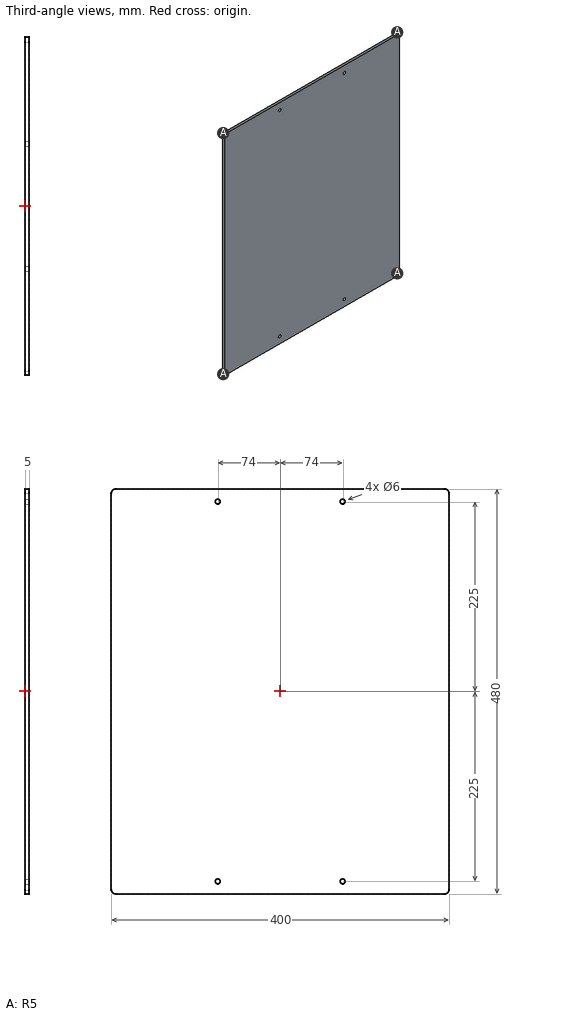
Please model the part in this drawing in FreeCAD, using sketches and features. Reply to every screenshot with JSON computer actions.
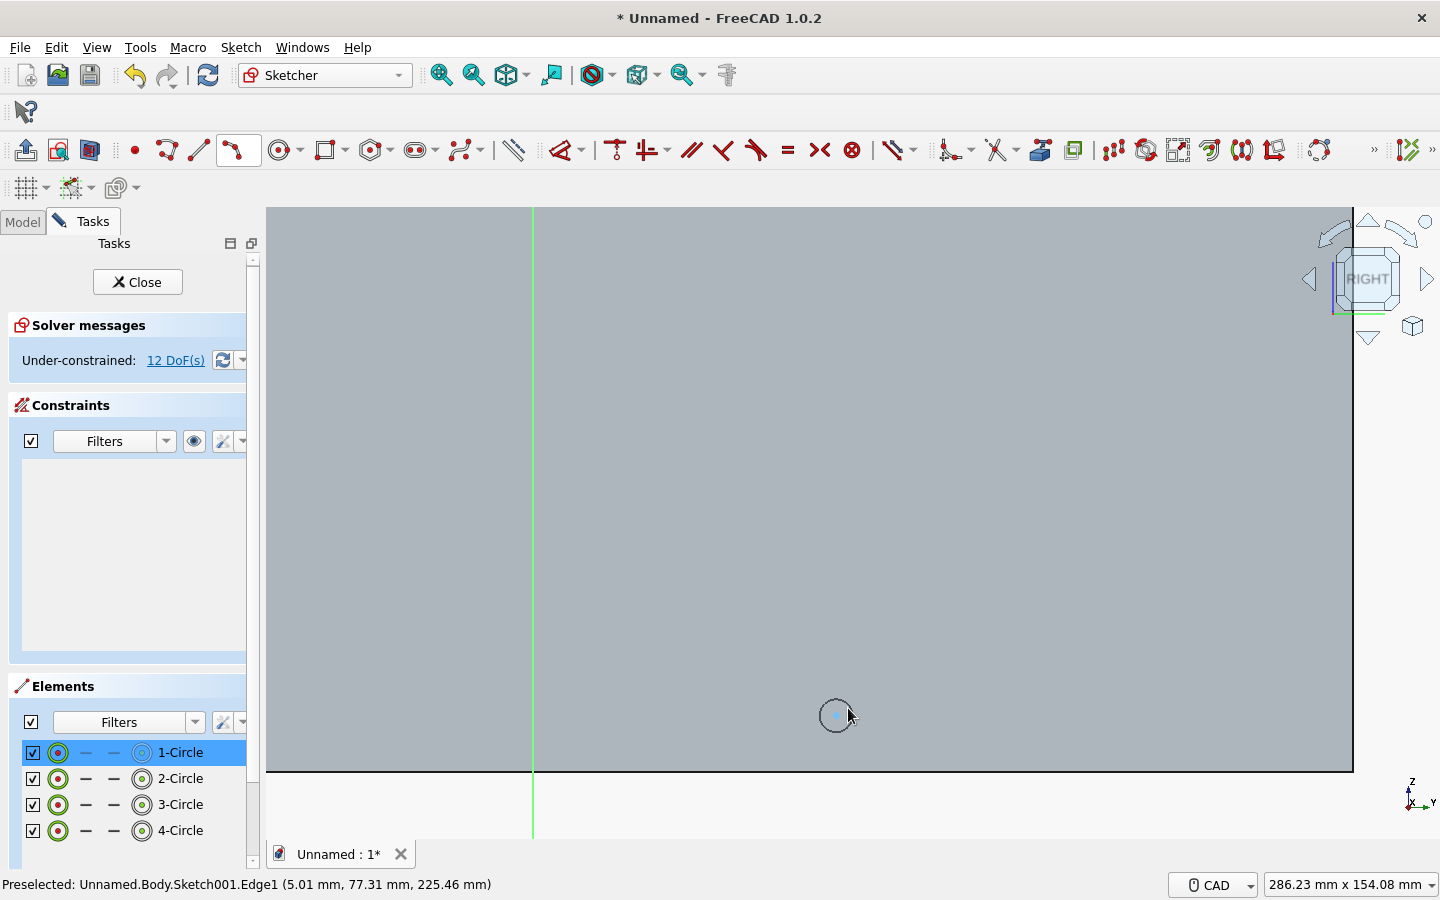
{"action": "left_click", "coordinate": [848, 704]}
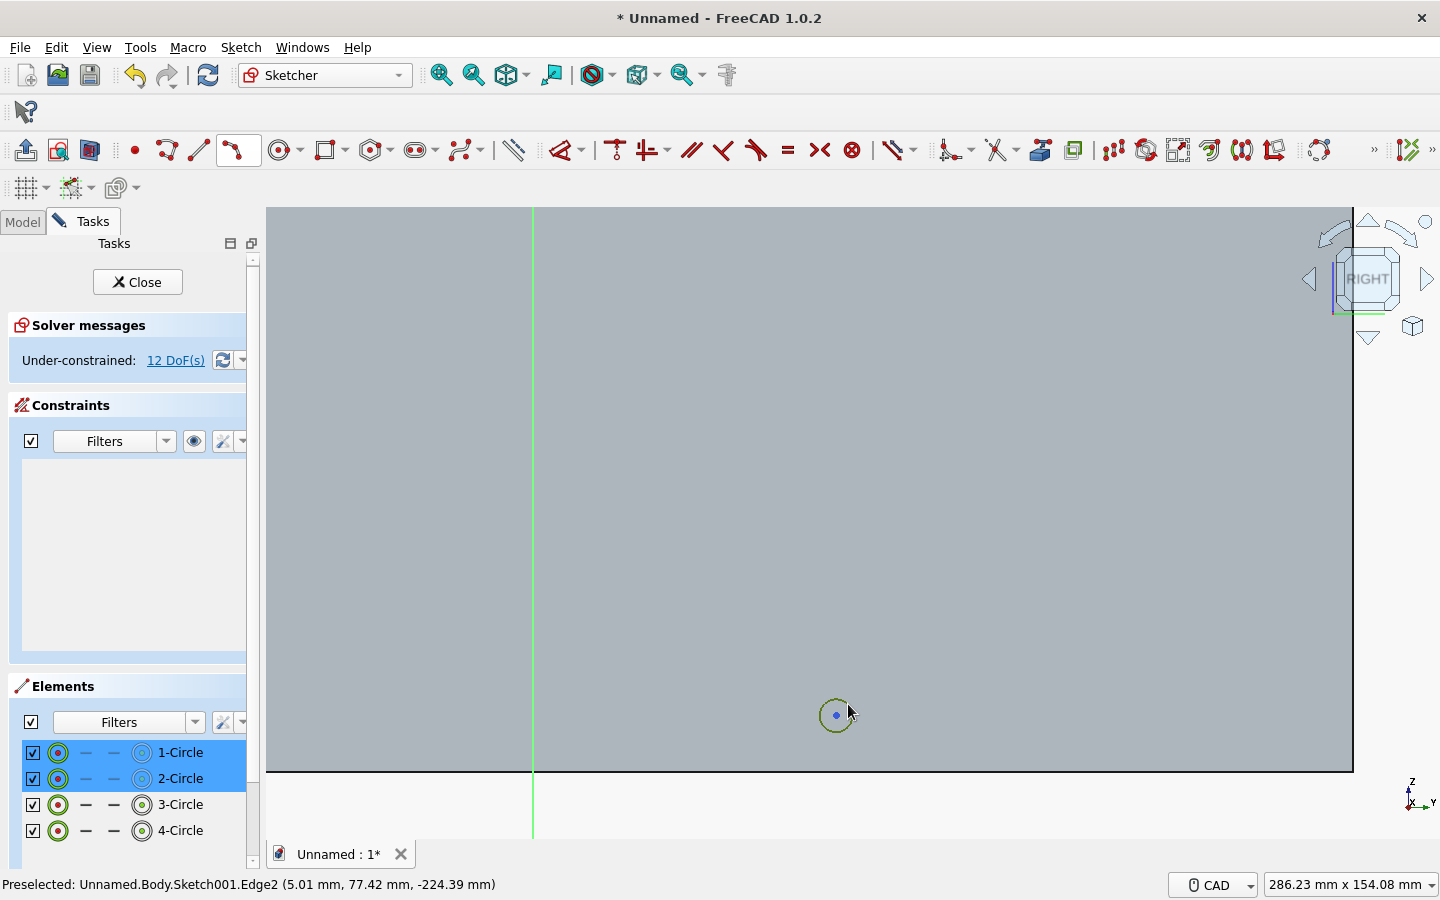
{"action": "scroll", "coordinate": [848, 709], "scroll_direction": "down", "scroll_amount": 8}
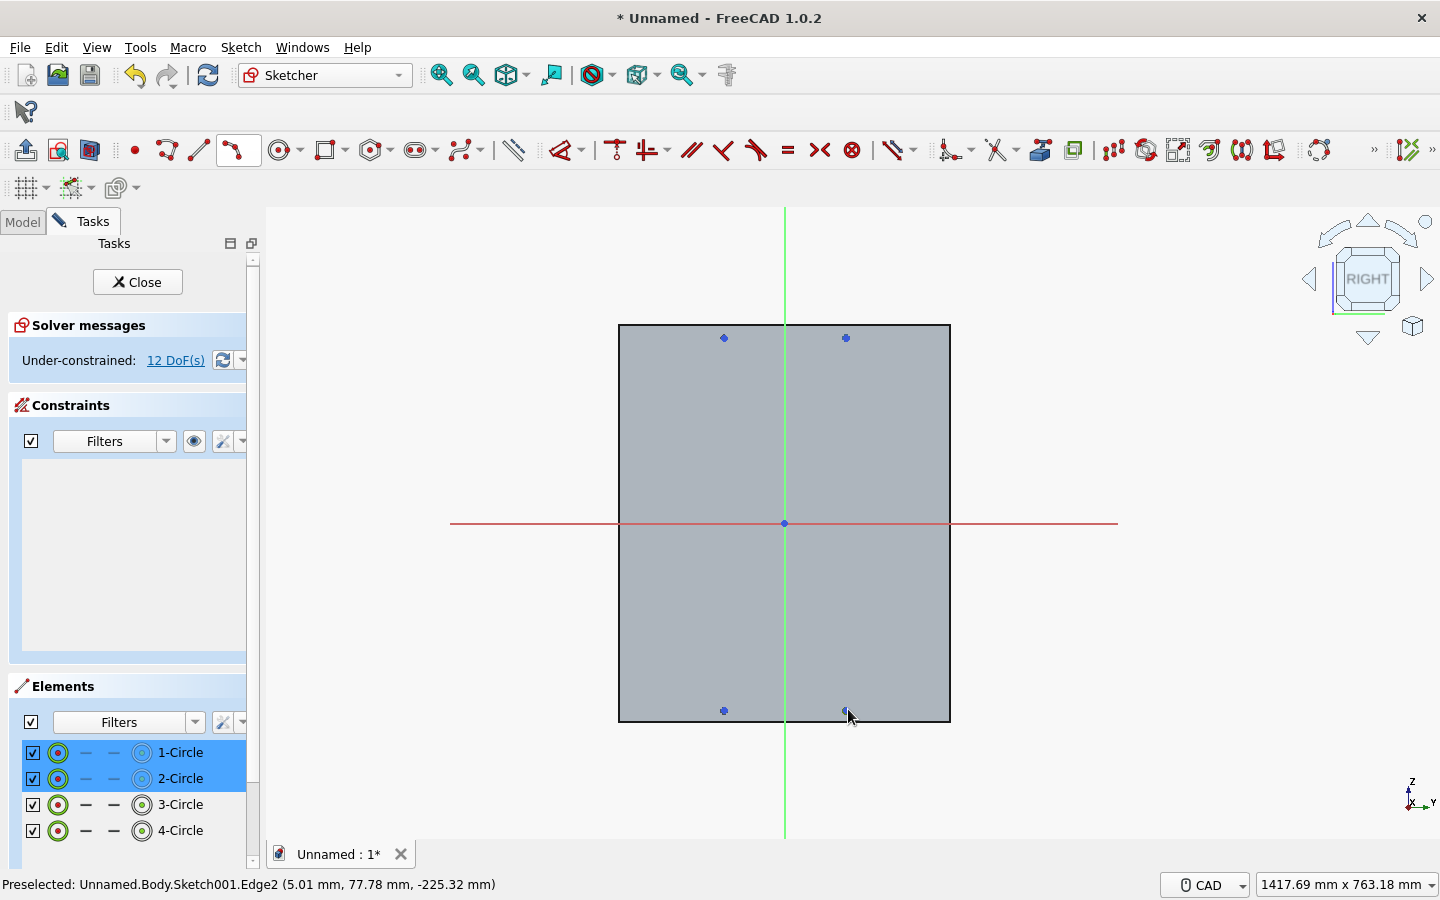
{"action": "scroll", "coordinate": [726, 336], "scroll_direction": "up", "scroll_amount": 9}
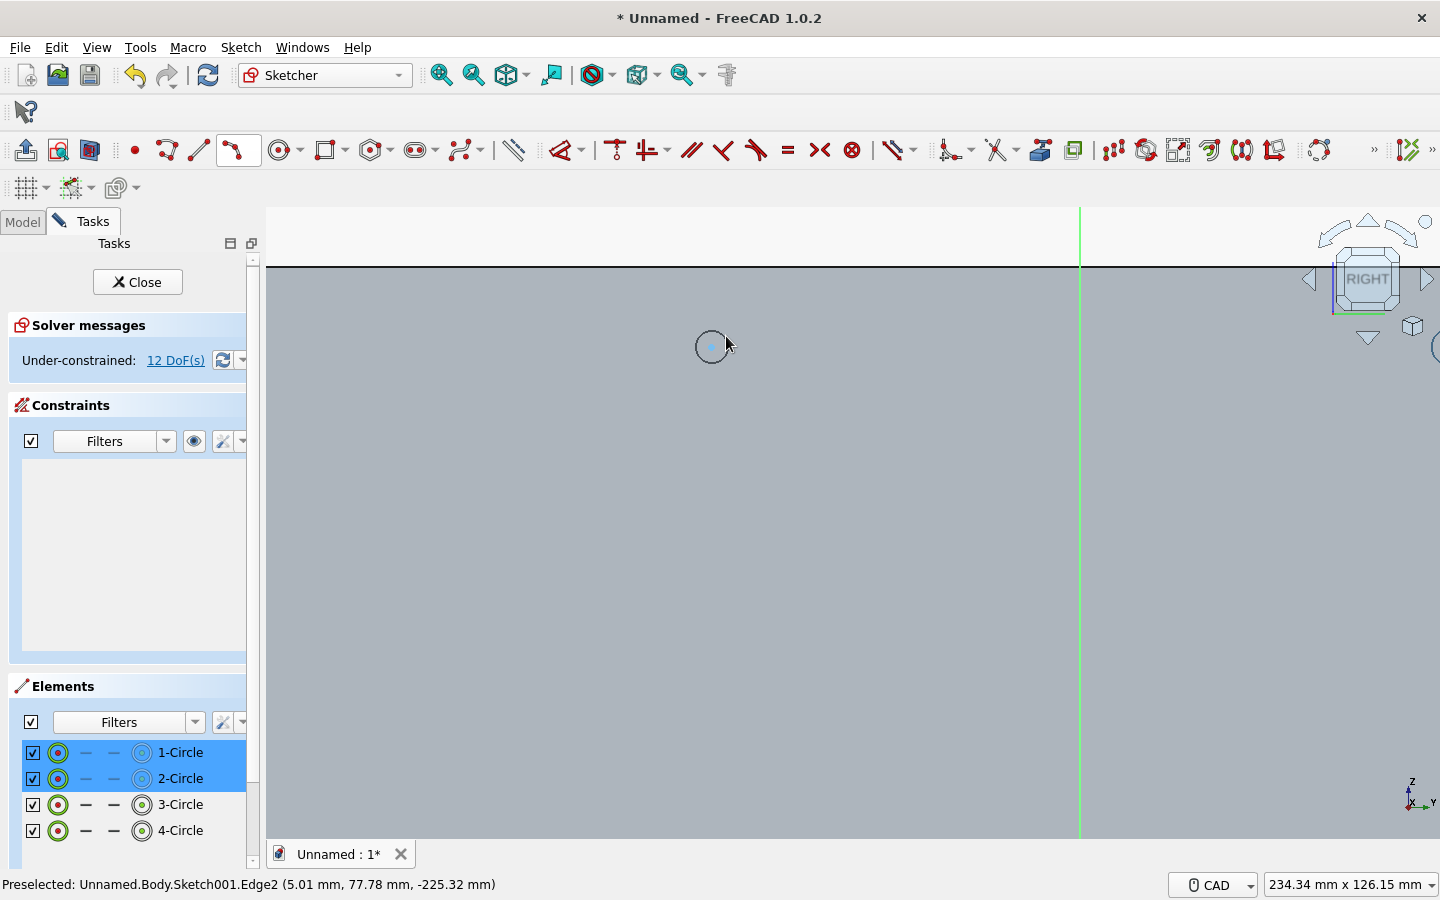
{"action": "left_click", "coordinate": [723, 336]}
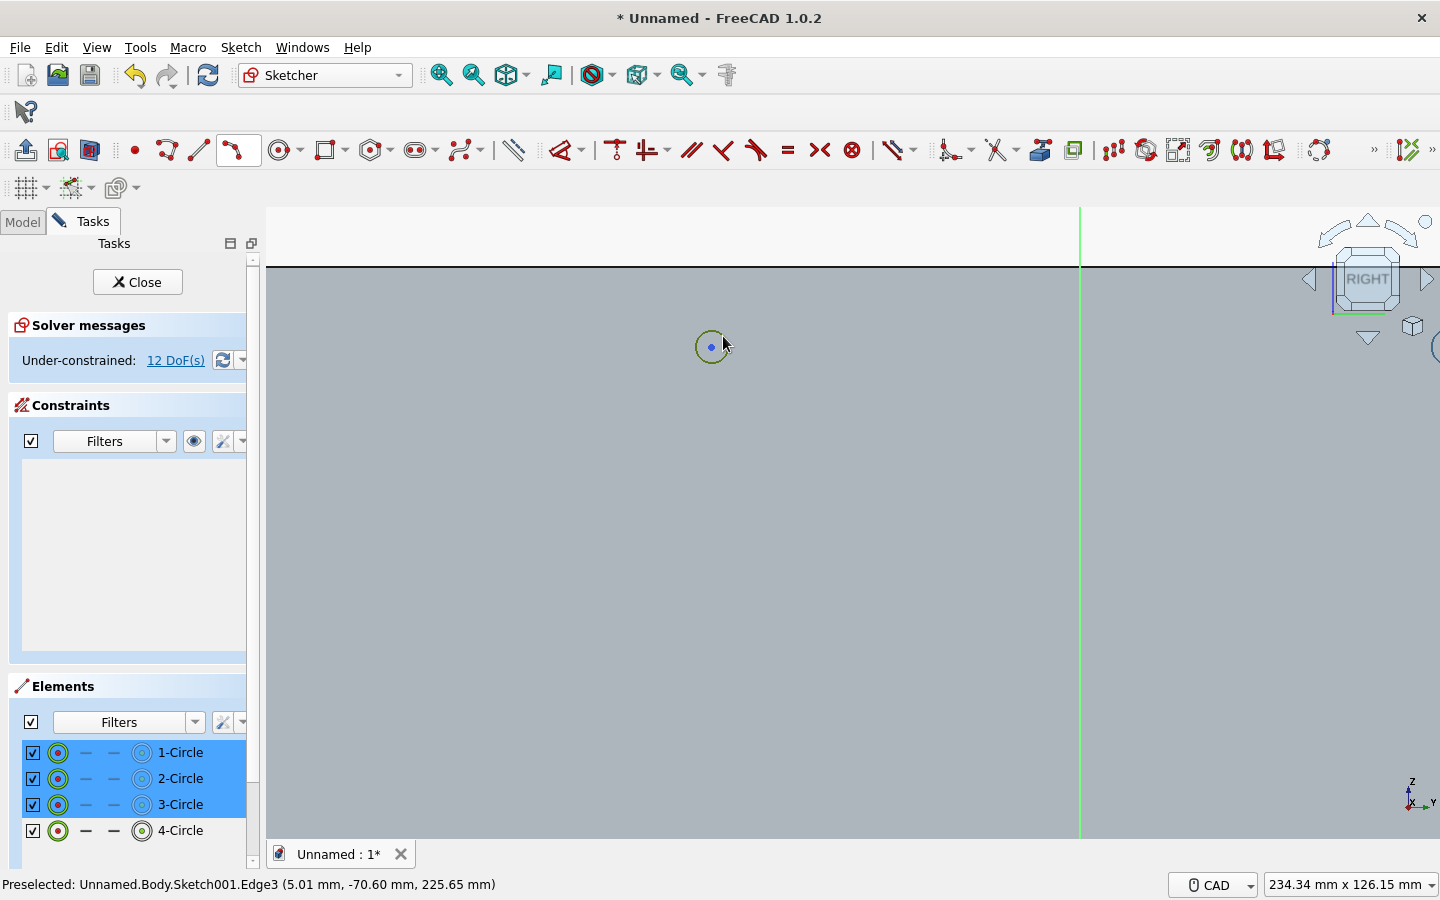
{"action": "scroll", "coordinate": [726, 335], "scroll_direction": "down", "scroll_amount": 9}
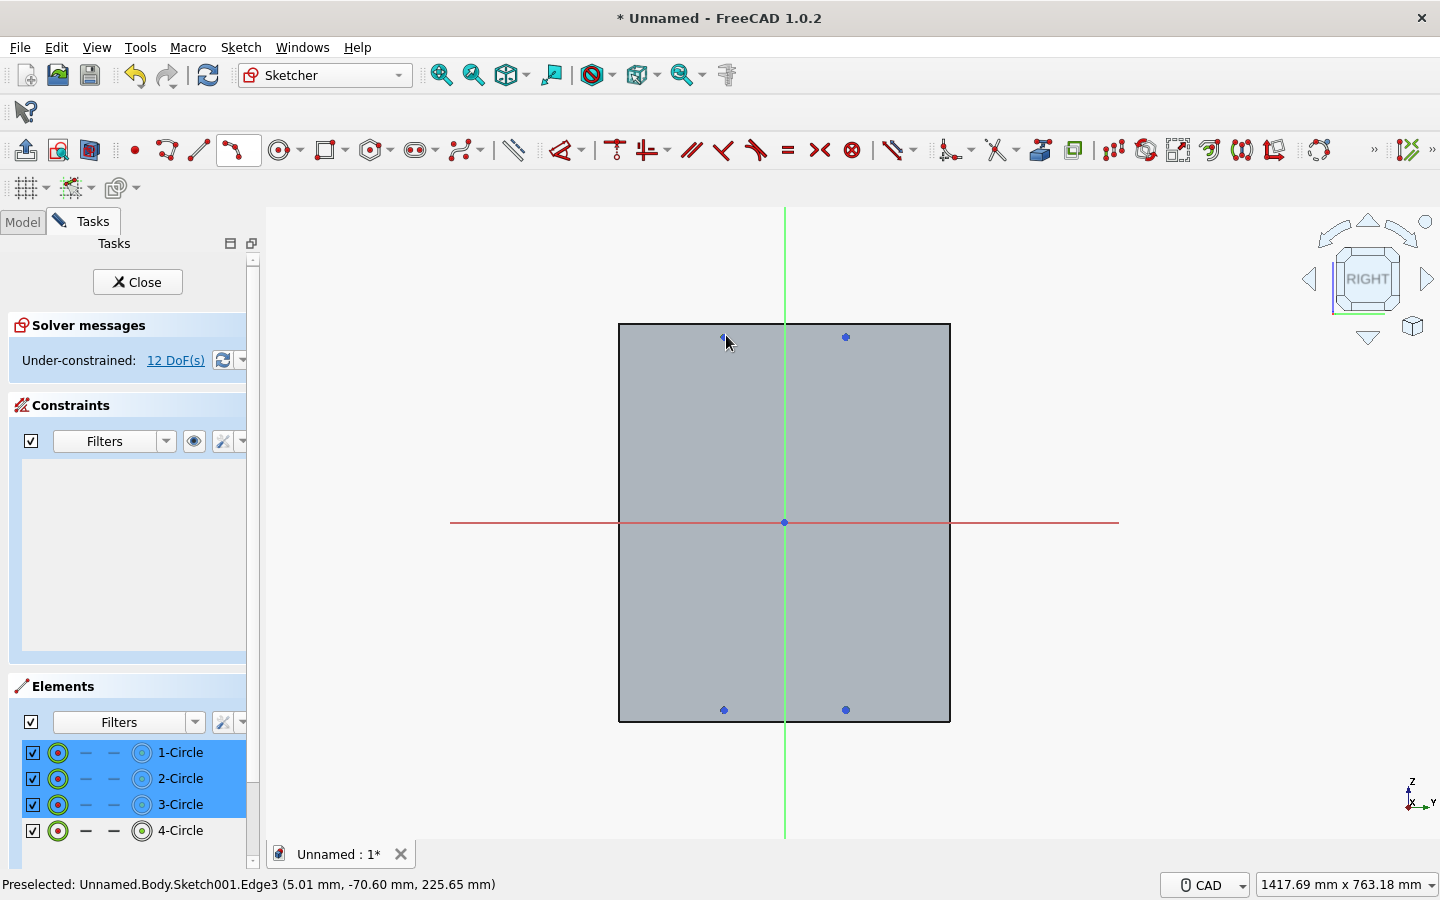
{"action": "scroll", "coordinate": [726, 708], "scroll_direction": "up", "scroll_amount": 8}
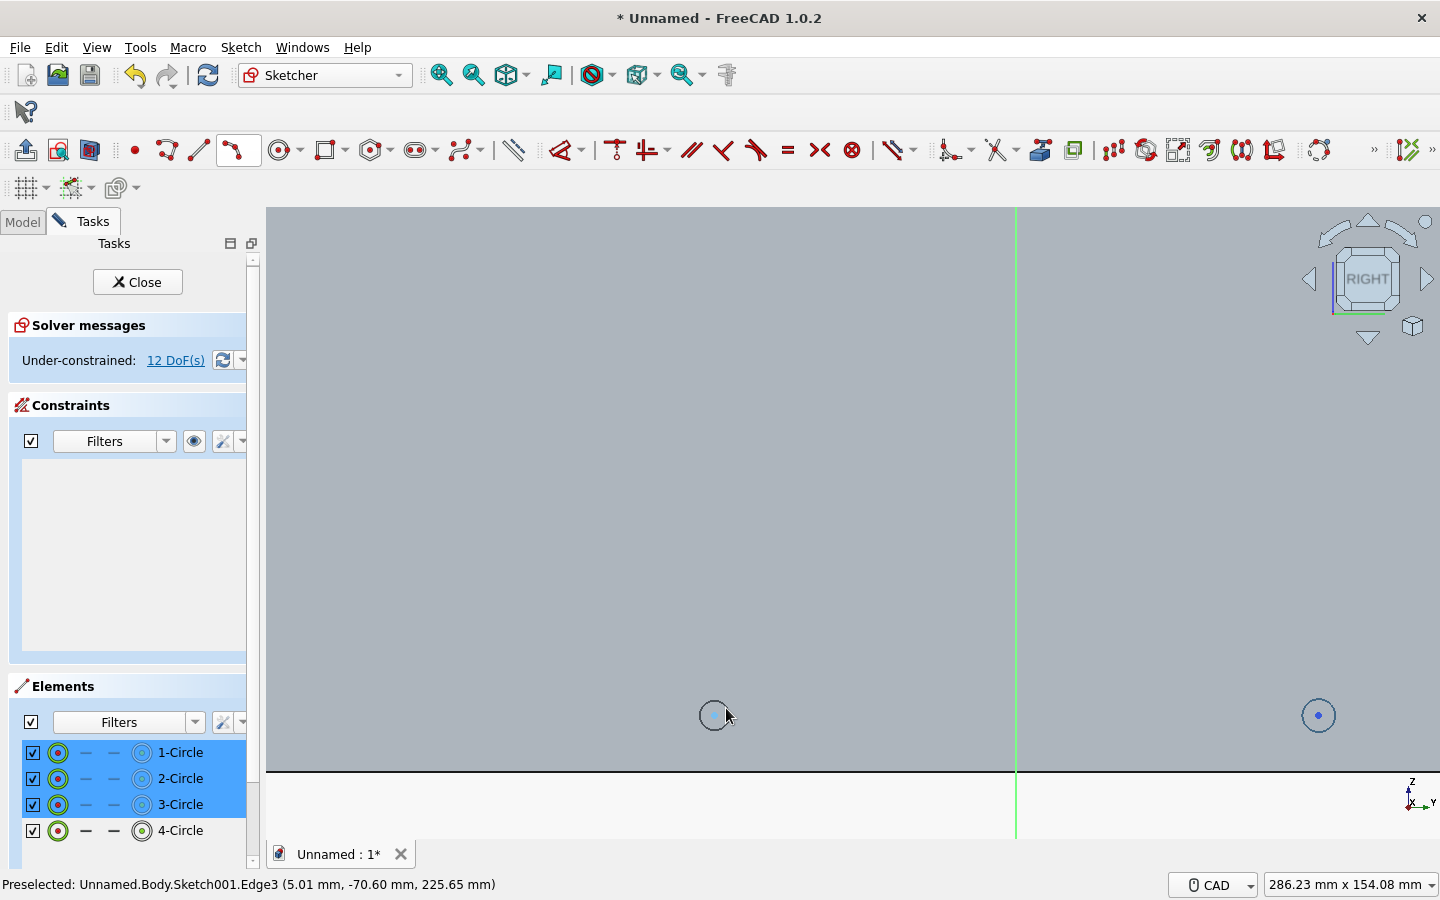
{"action": "left_click", "coordinate": [725, 705]}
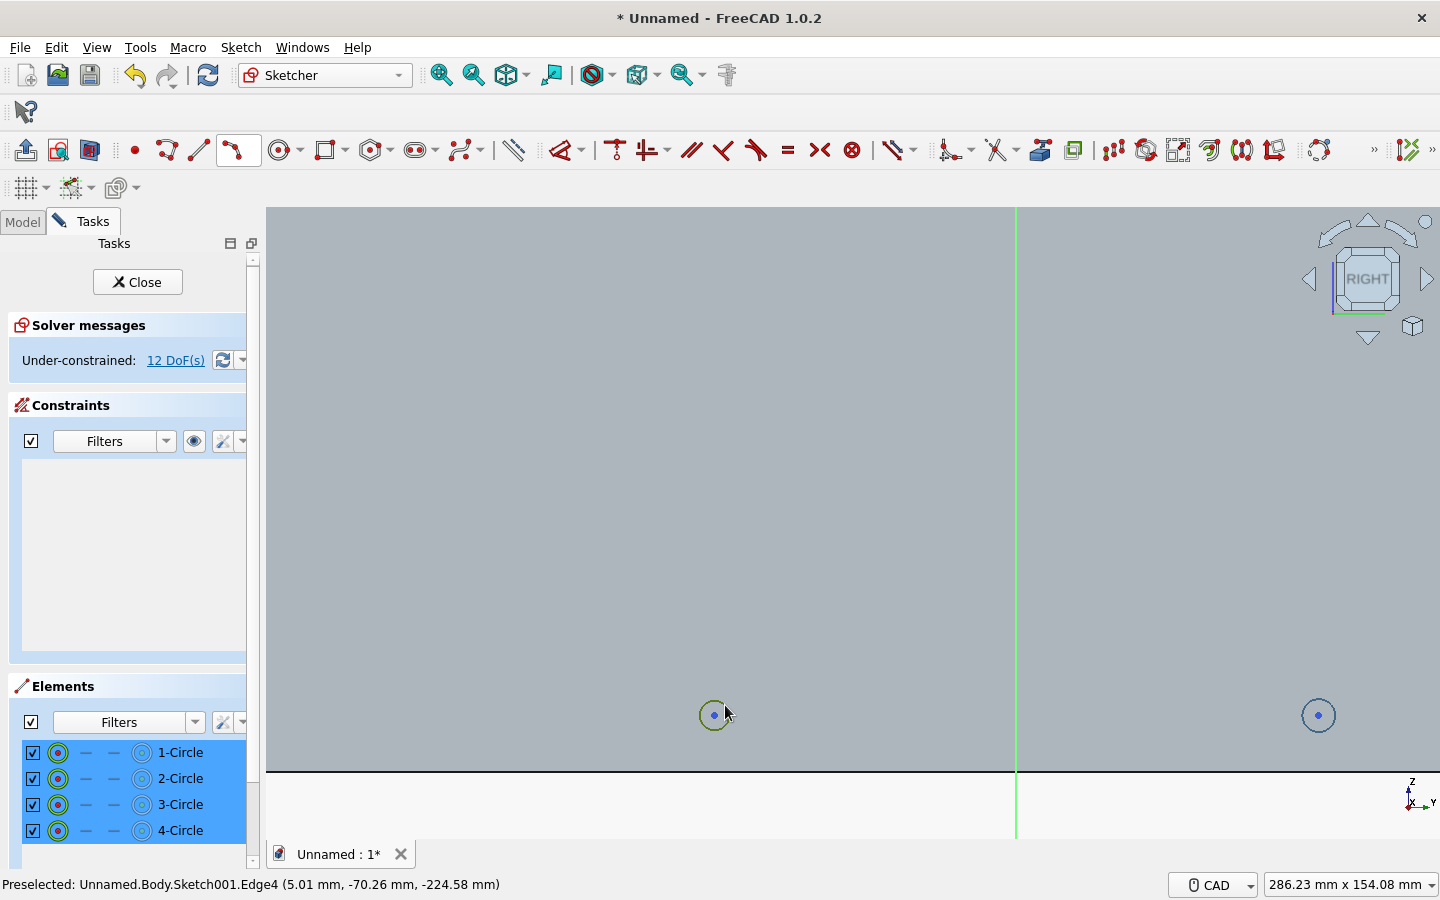
{"action": "key", "text": "e"}